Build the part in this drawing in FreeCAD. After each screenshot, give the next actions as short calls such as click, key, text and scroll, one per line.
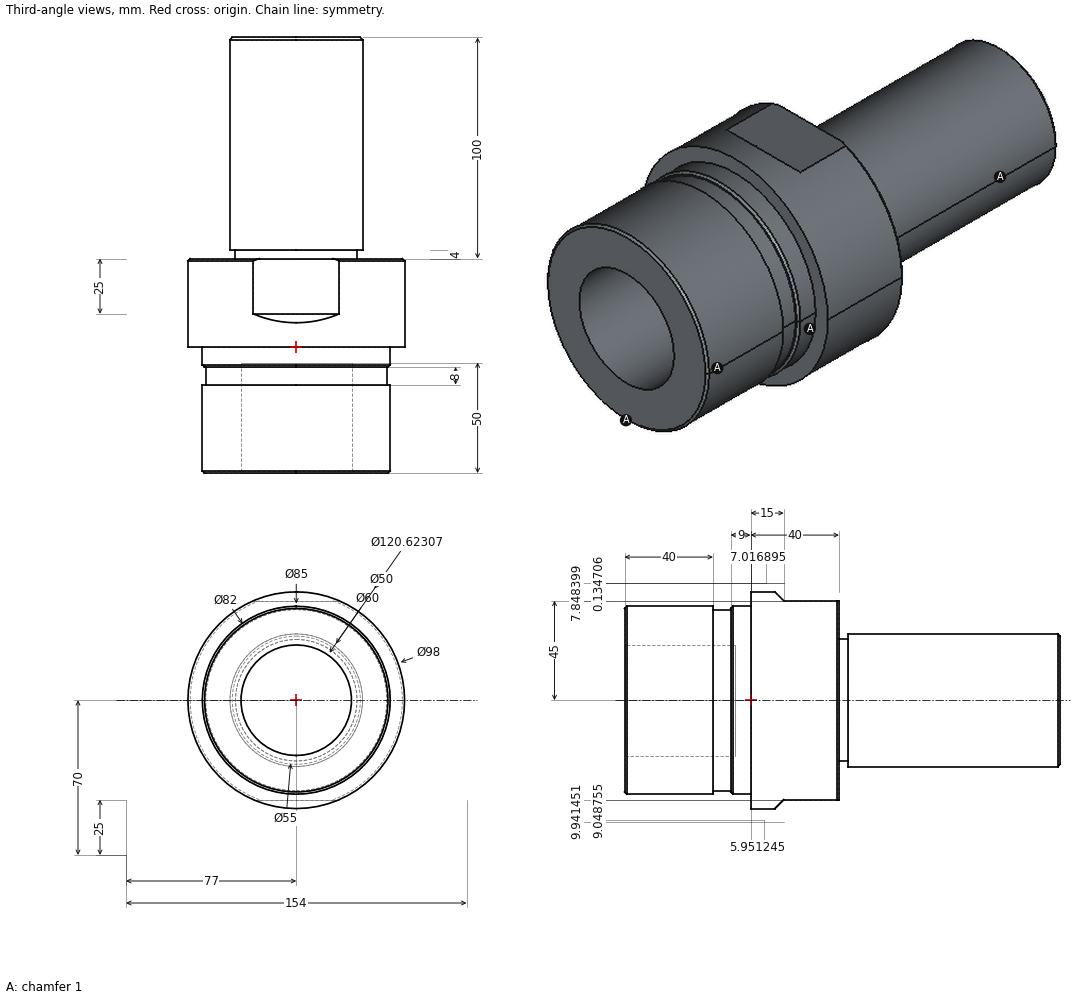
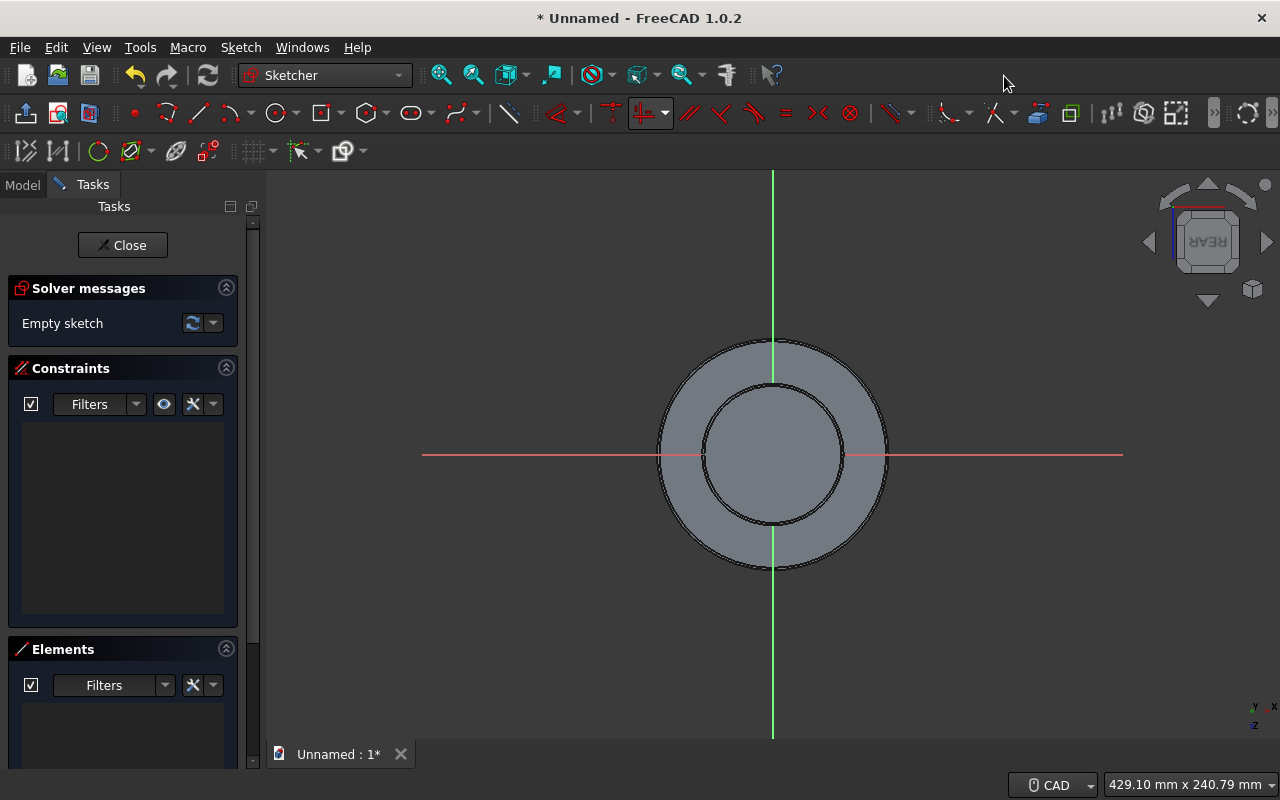
key(g)
key(r)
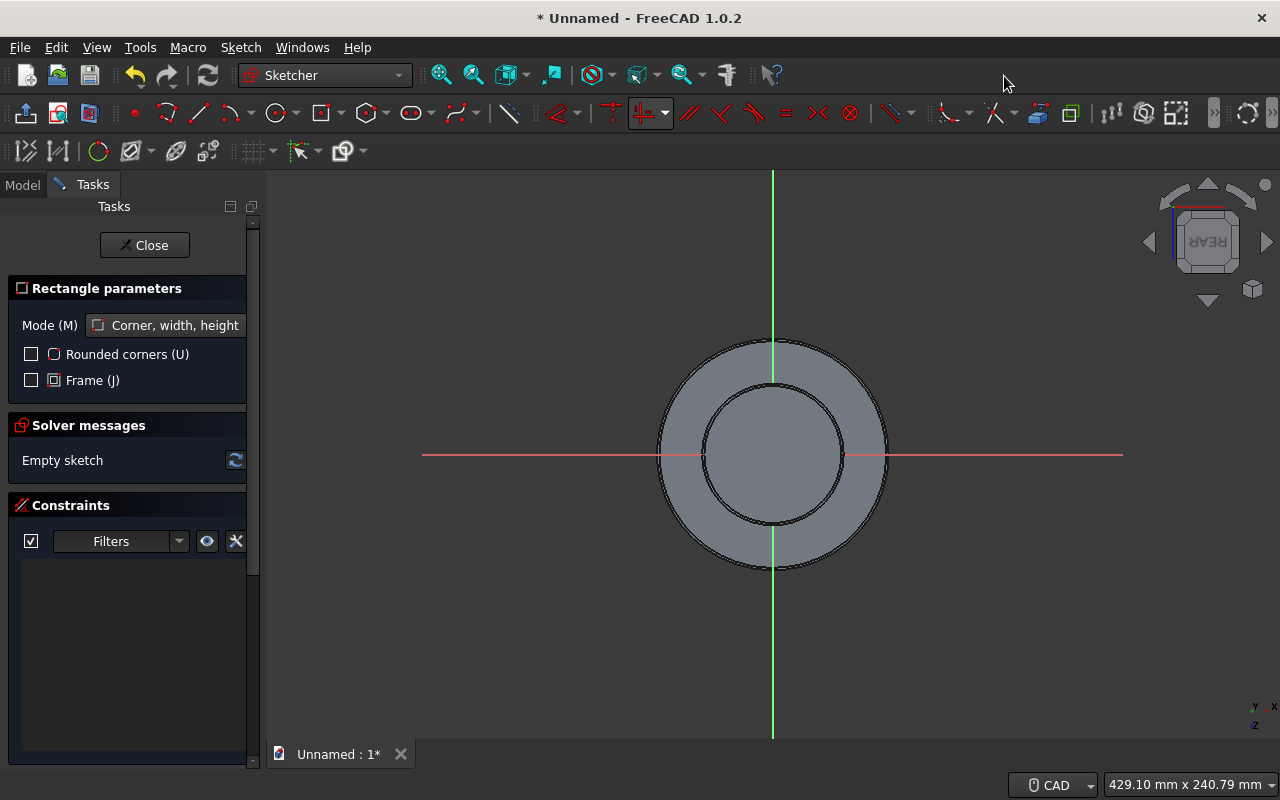
click(591, 289)
click(955, 348)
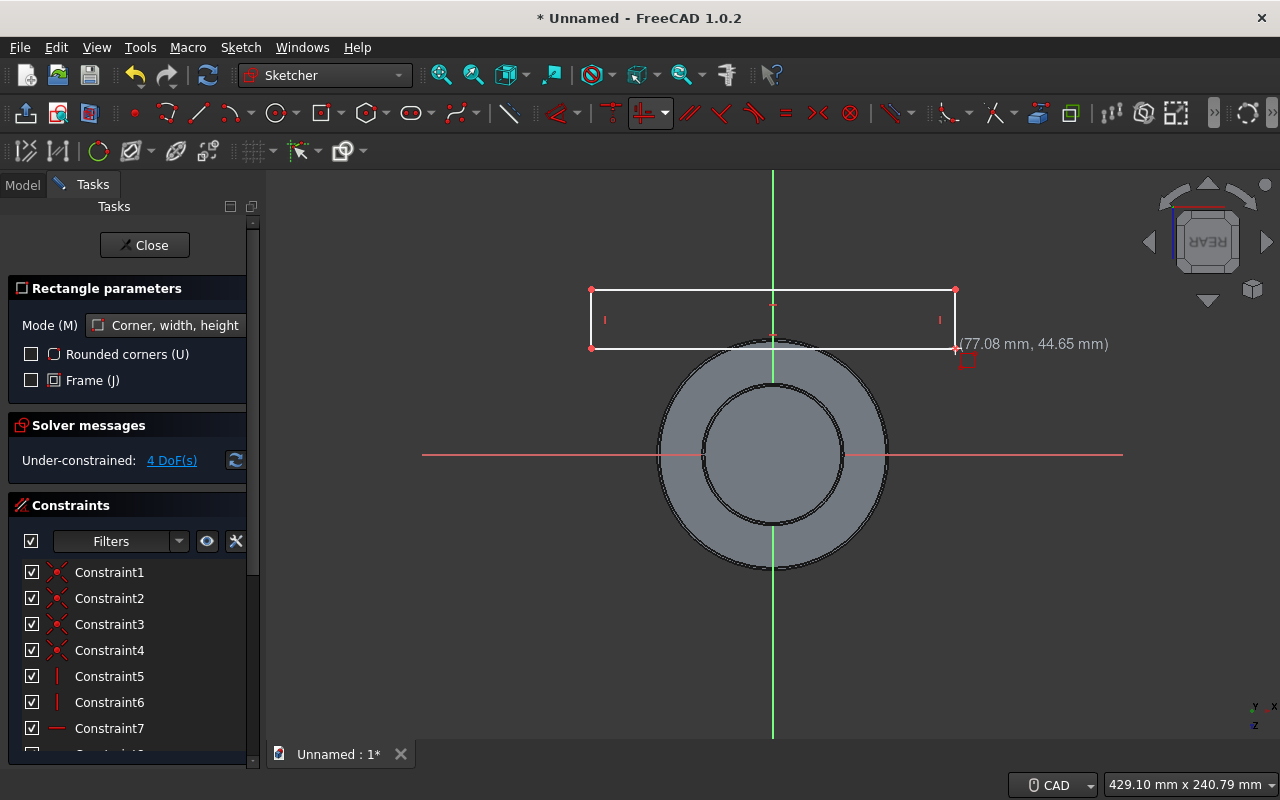
click(591, 561)
click(955, 620)
key(Escape)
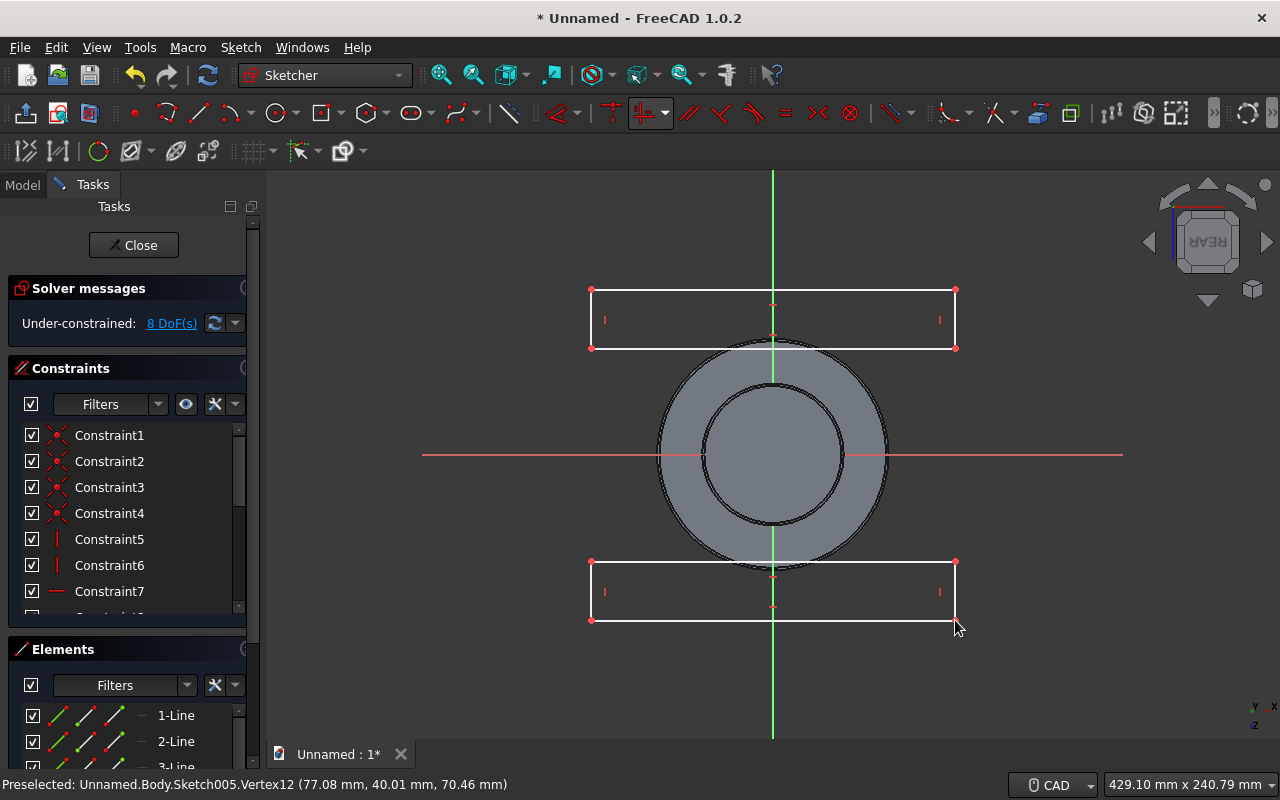
click(591, 349)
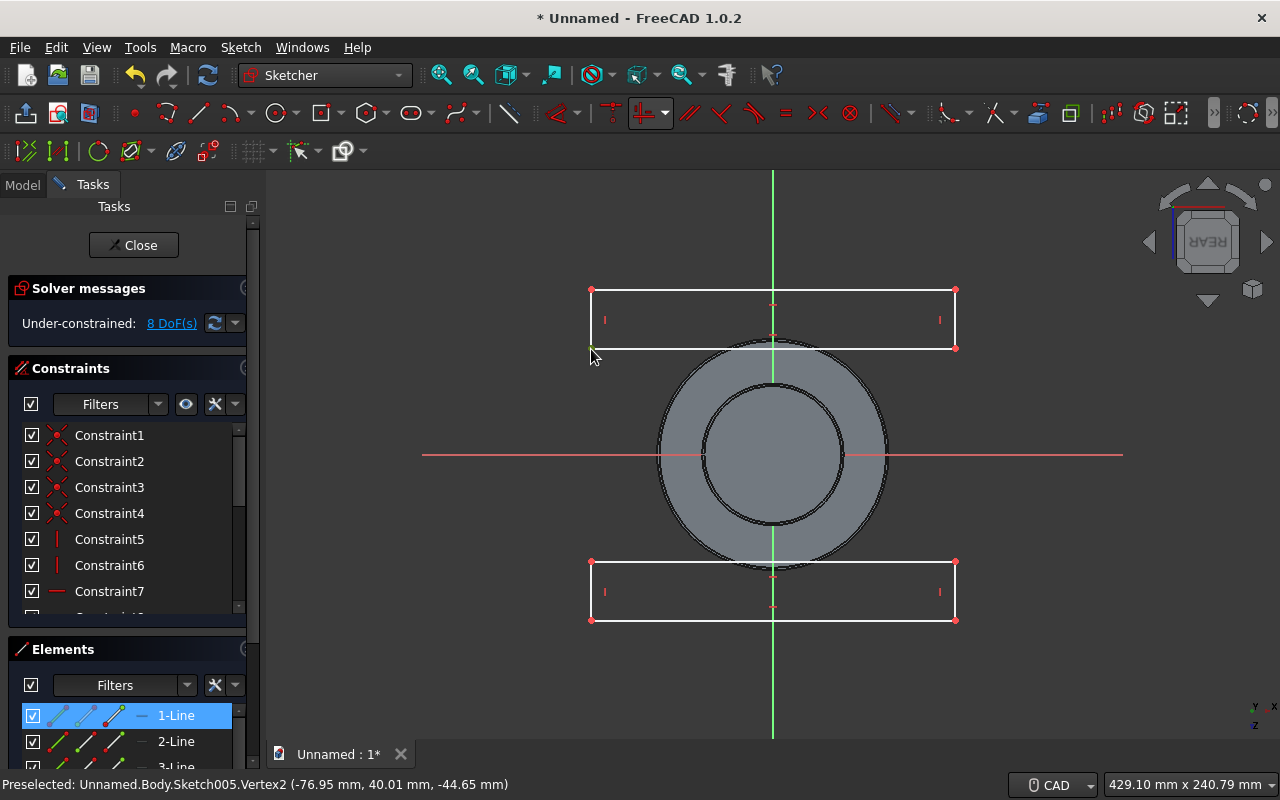
click(591, 562)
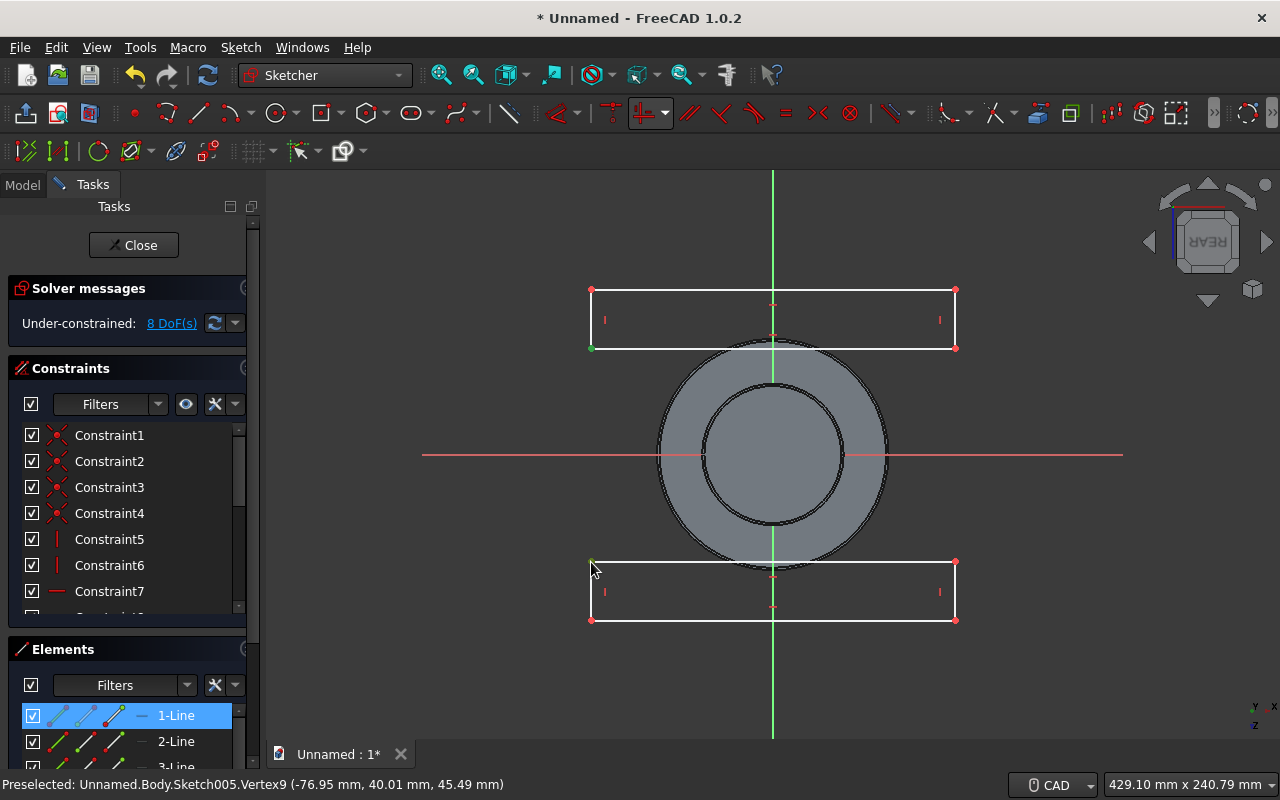
click(470, 454)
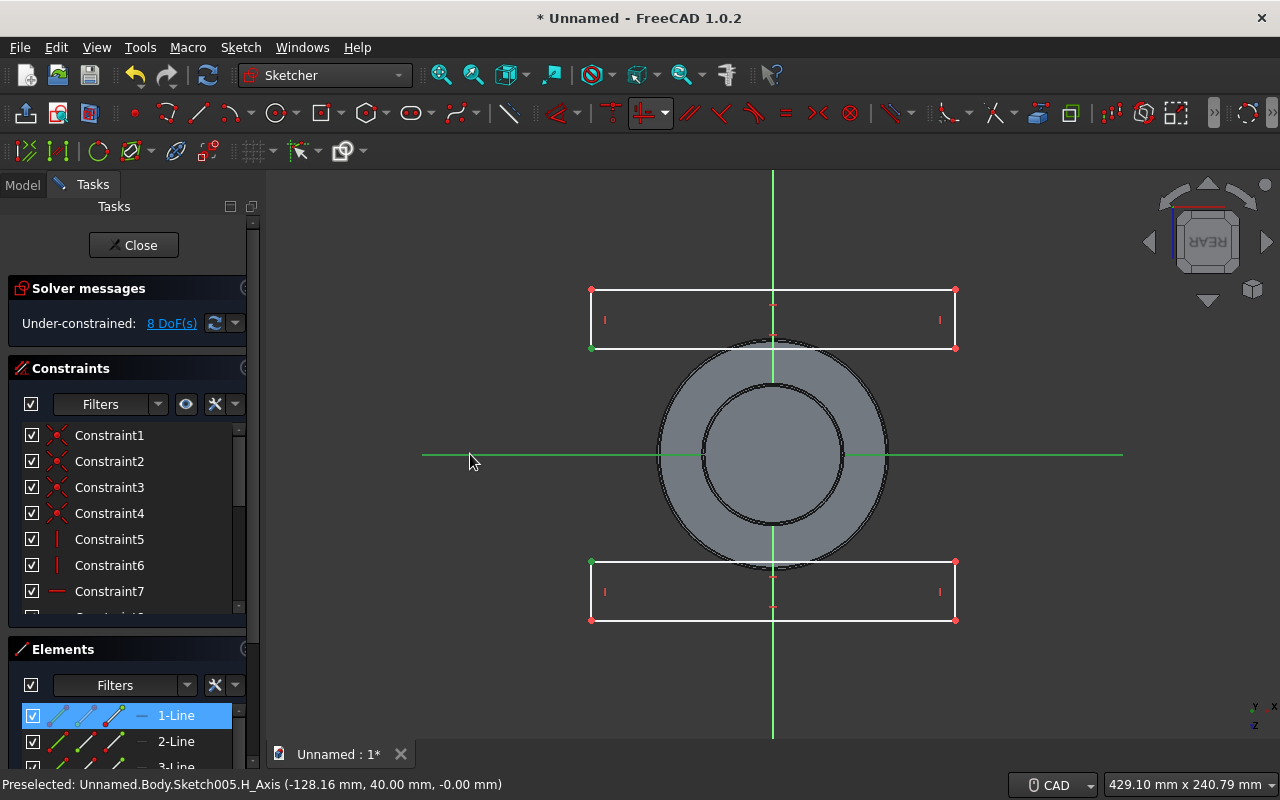
click(818, 114)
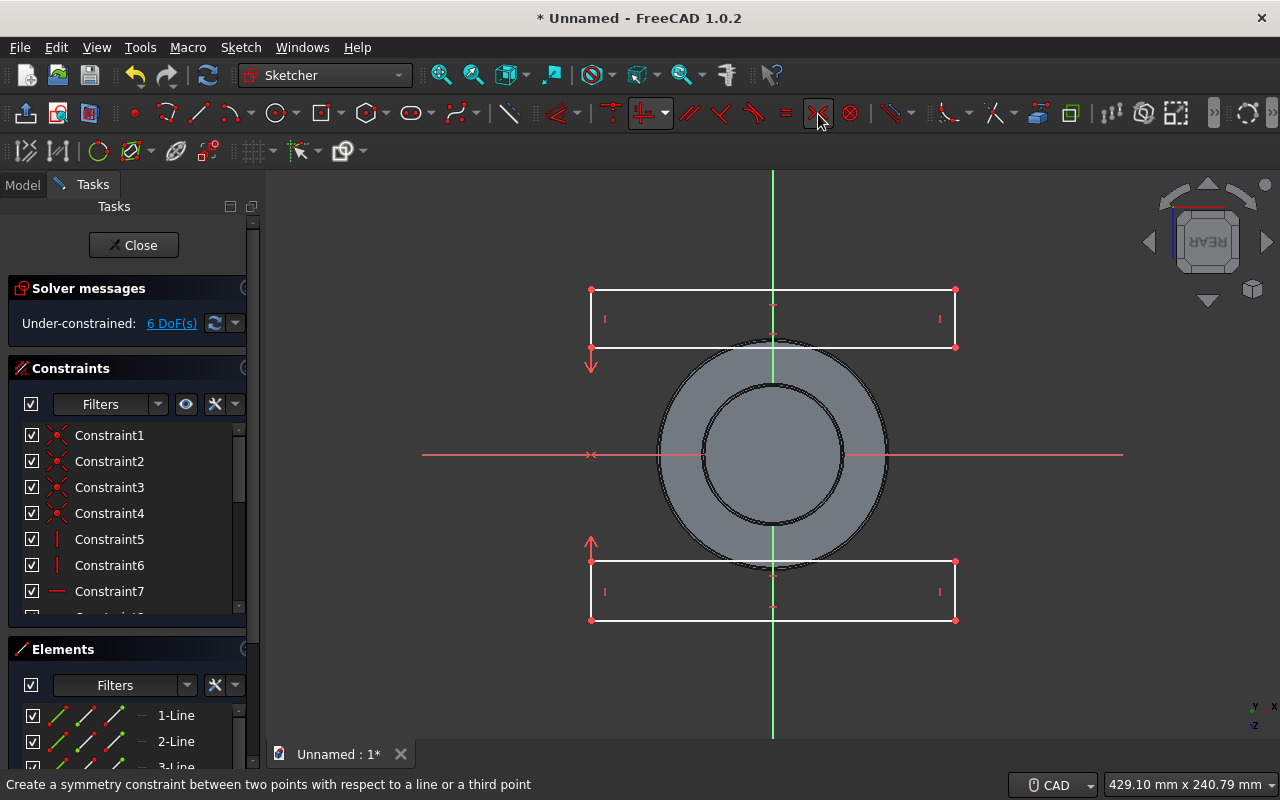
click(955, 290)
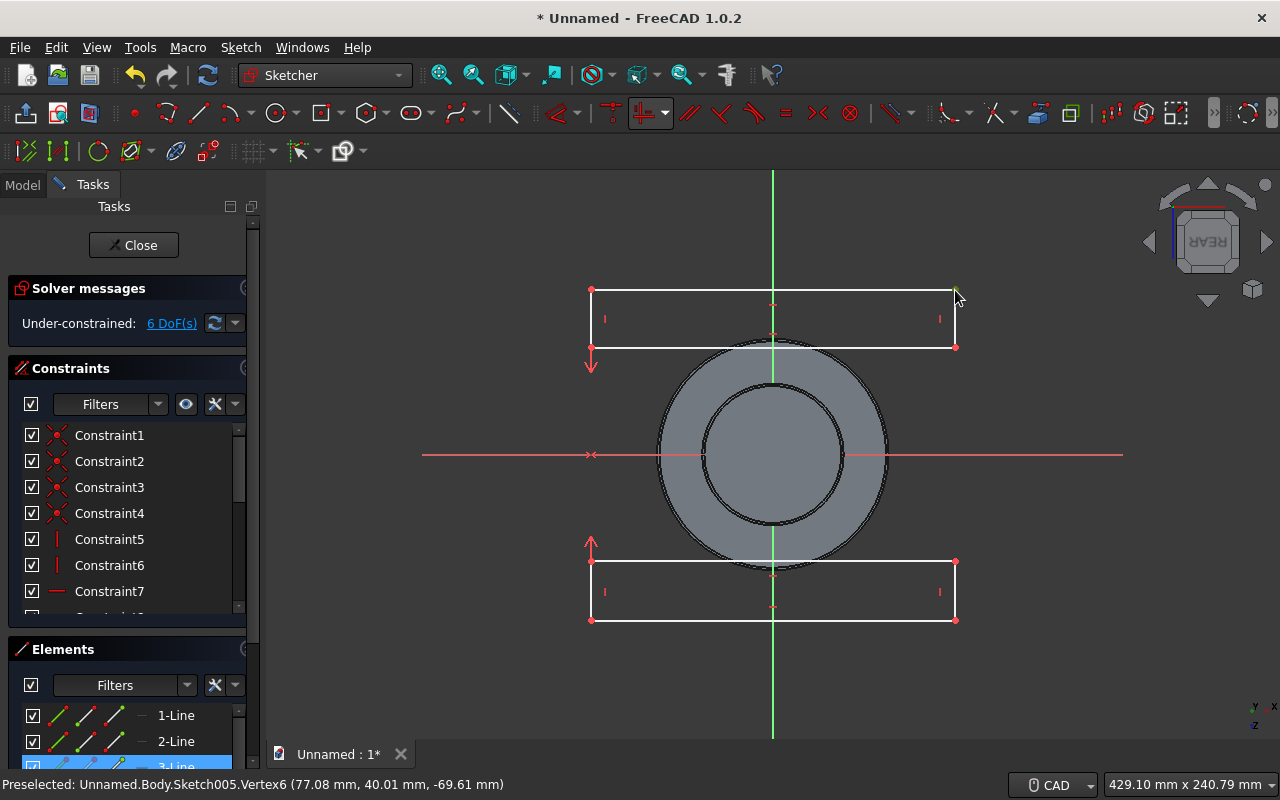
click(955, 621)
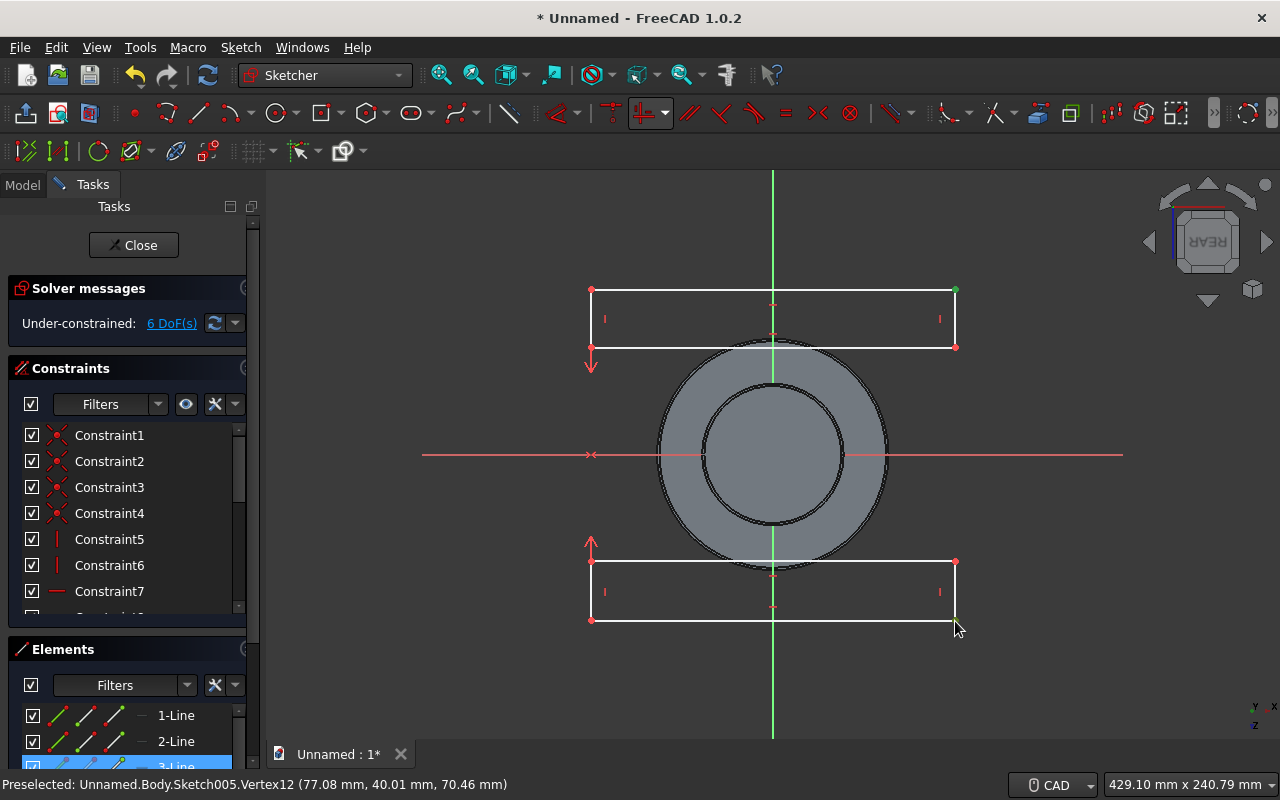
click(470, 454)